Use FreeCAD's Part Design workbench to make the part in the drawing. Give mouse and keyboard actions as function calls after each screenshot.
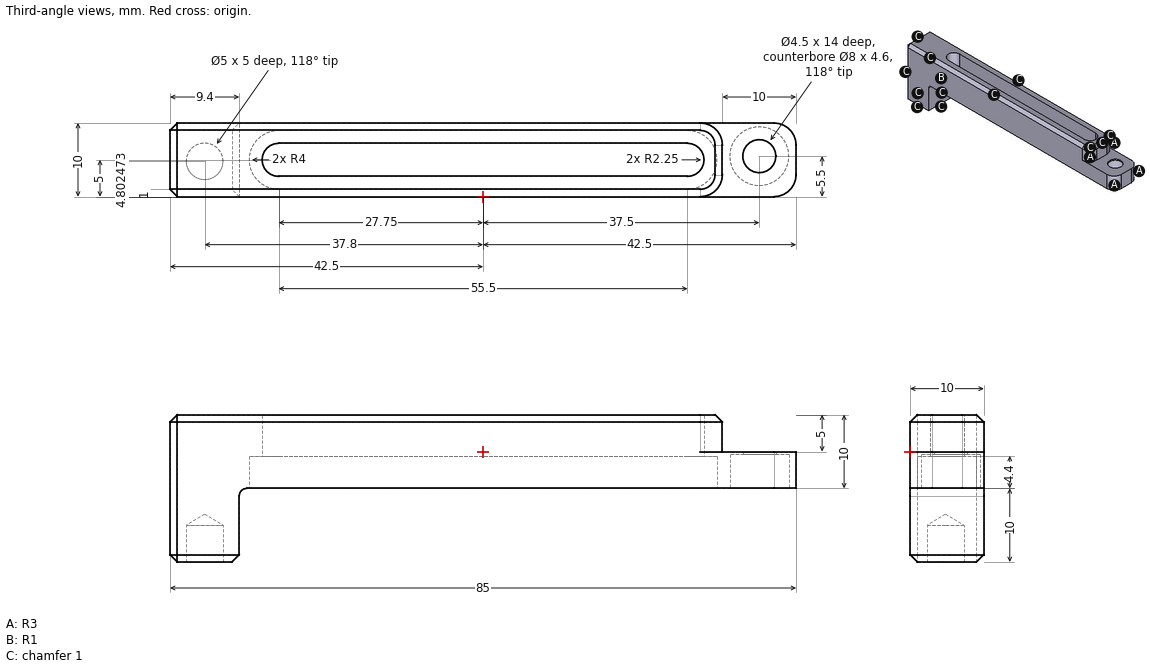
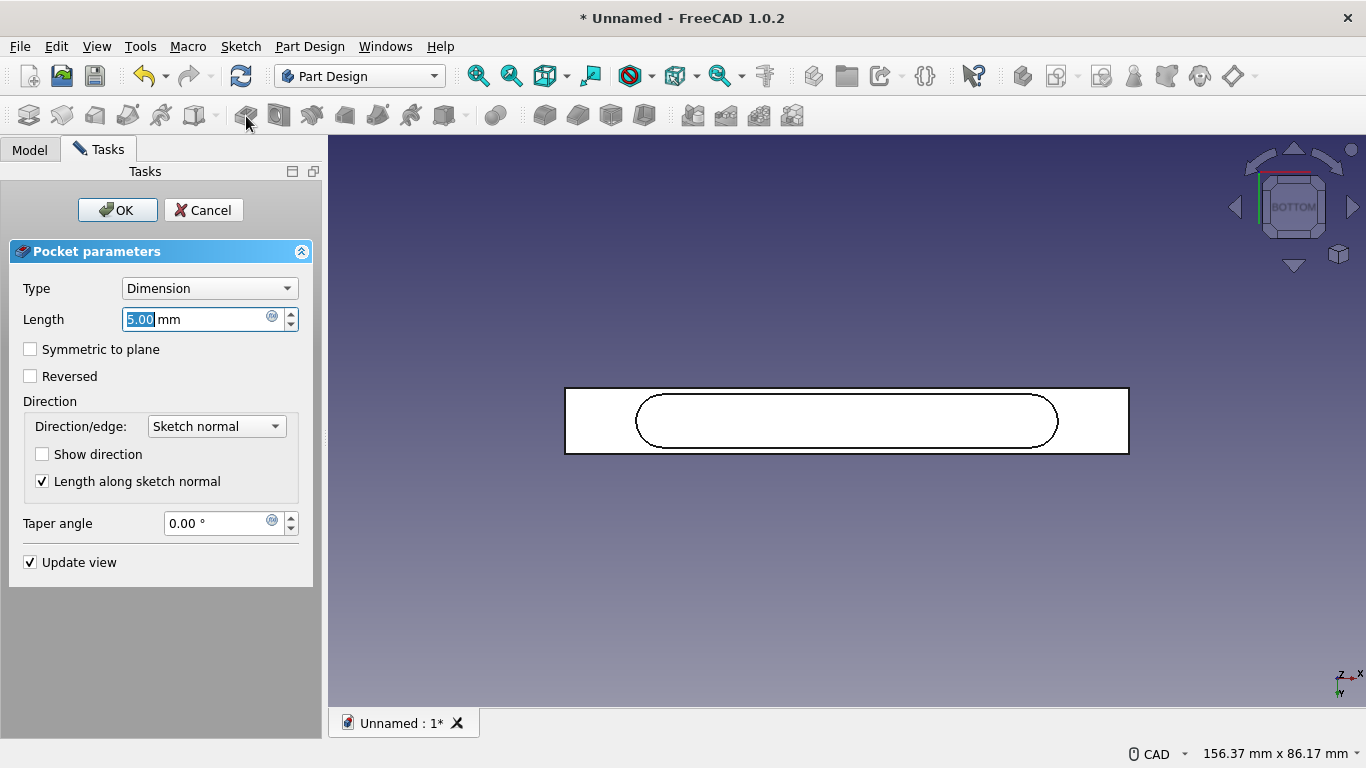
text(4.4)
key(Tab)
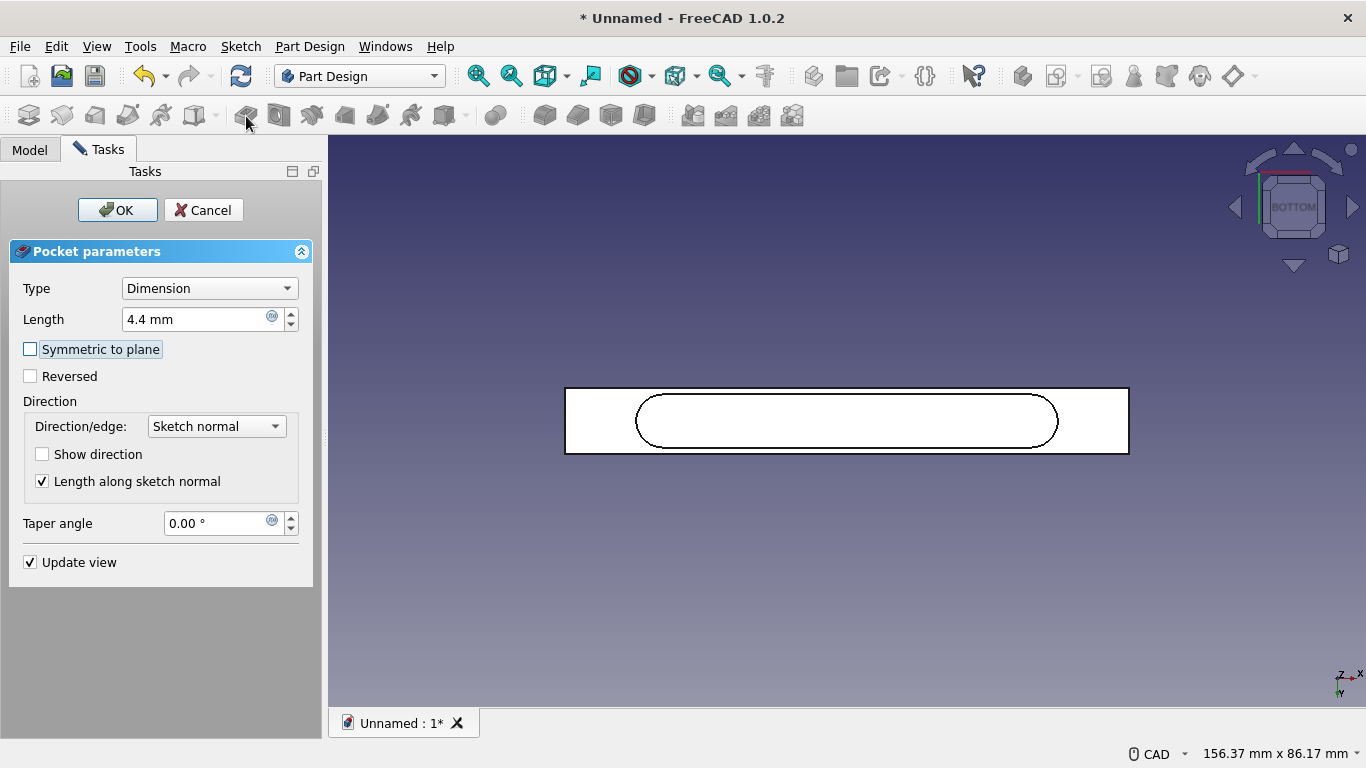
click(118, 210)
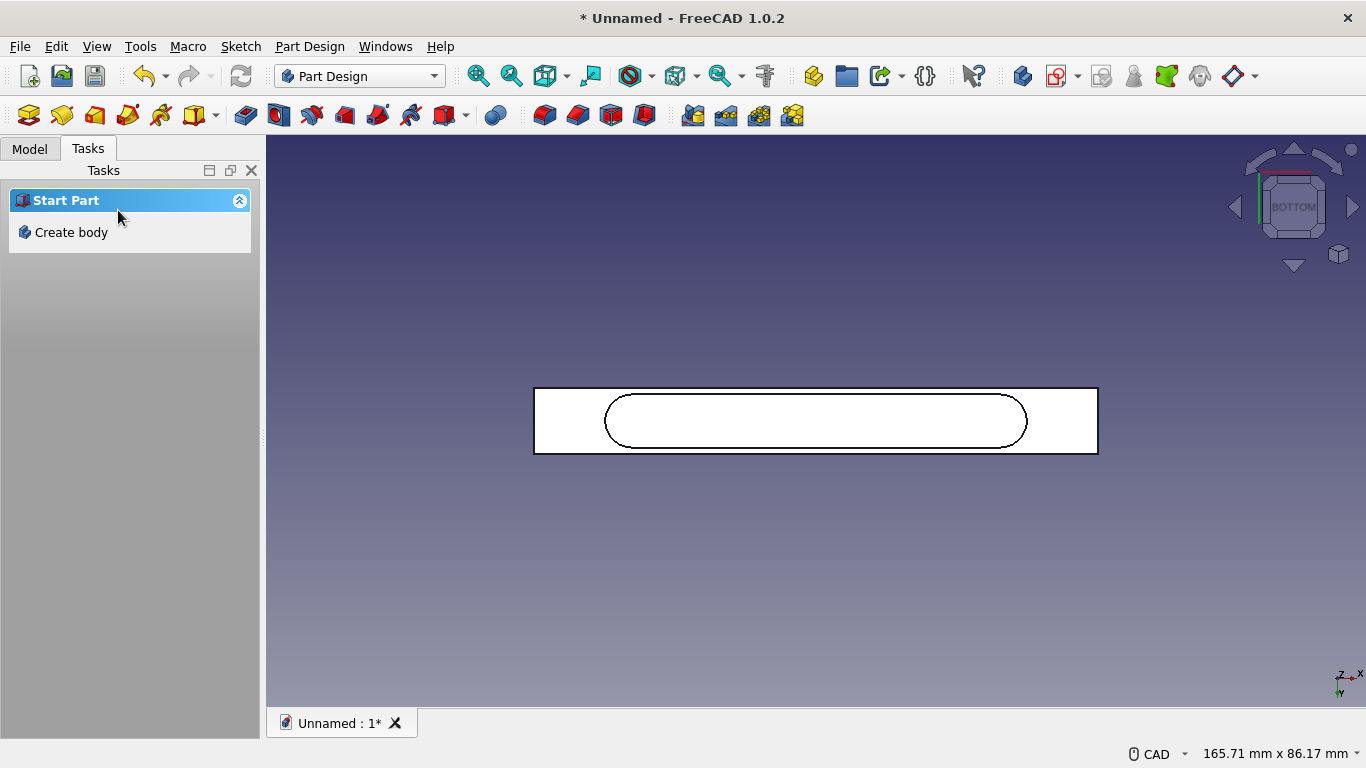
click(997, 420)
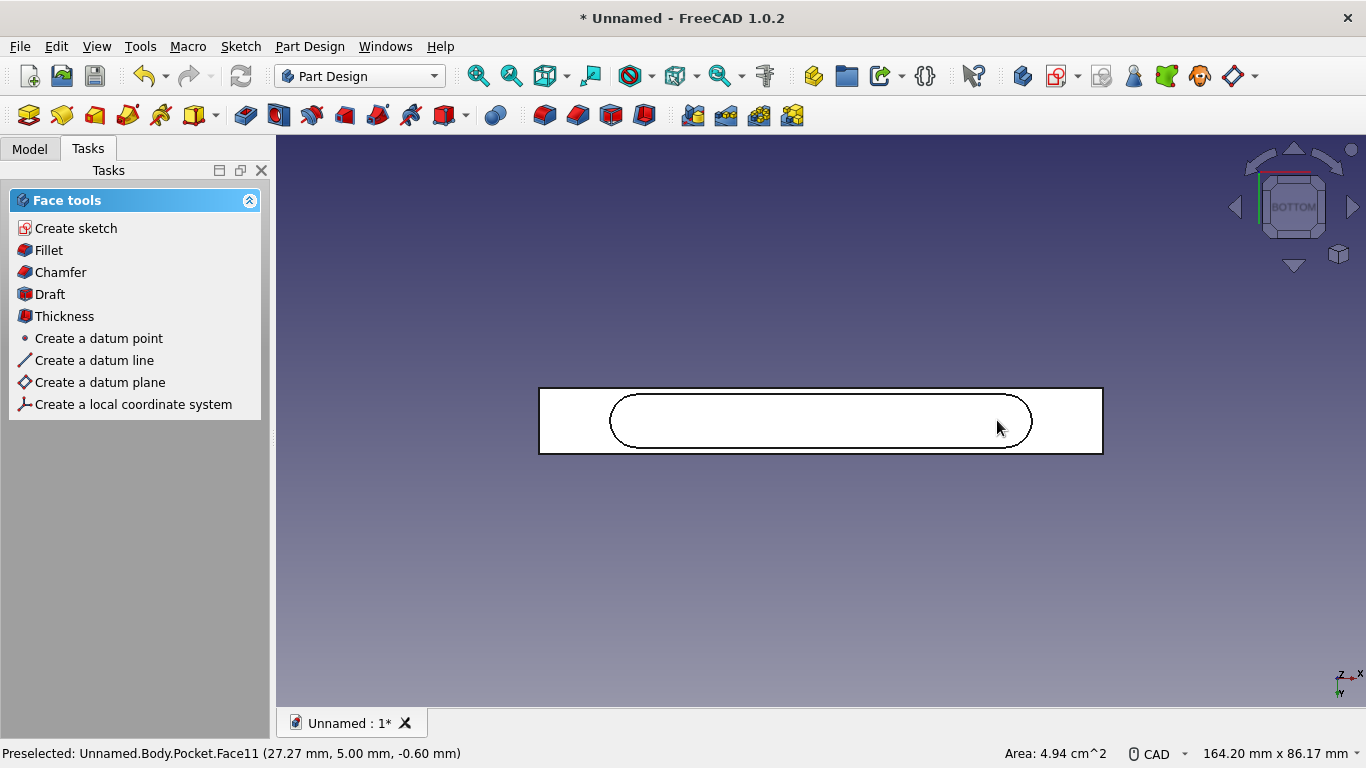
click(1056, 76)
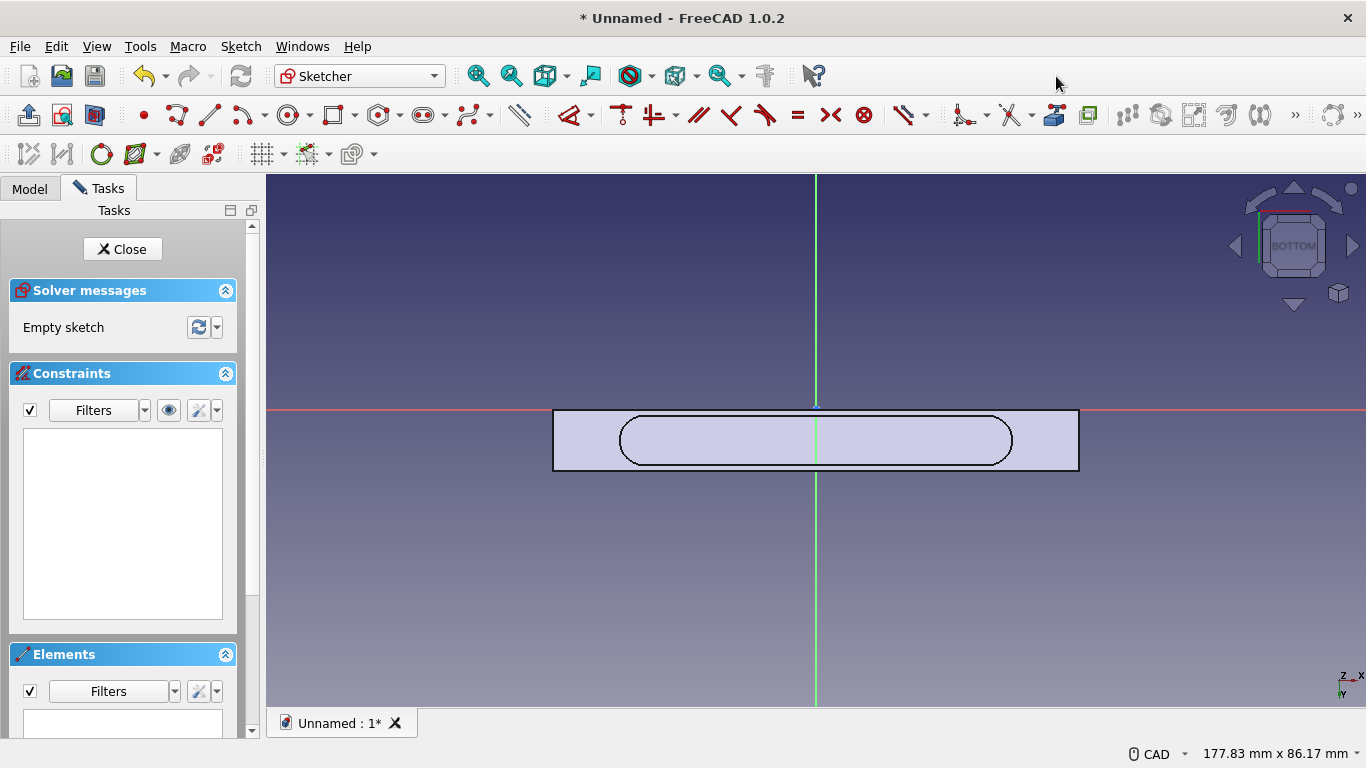
scroll(899, 422, up, 3)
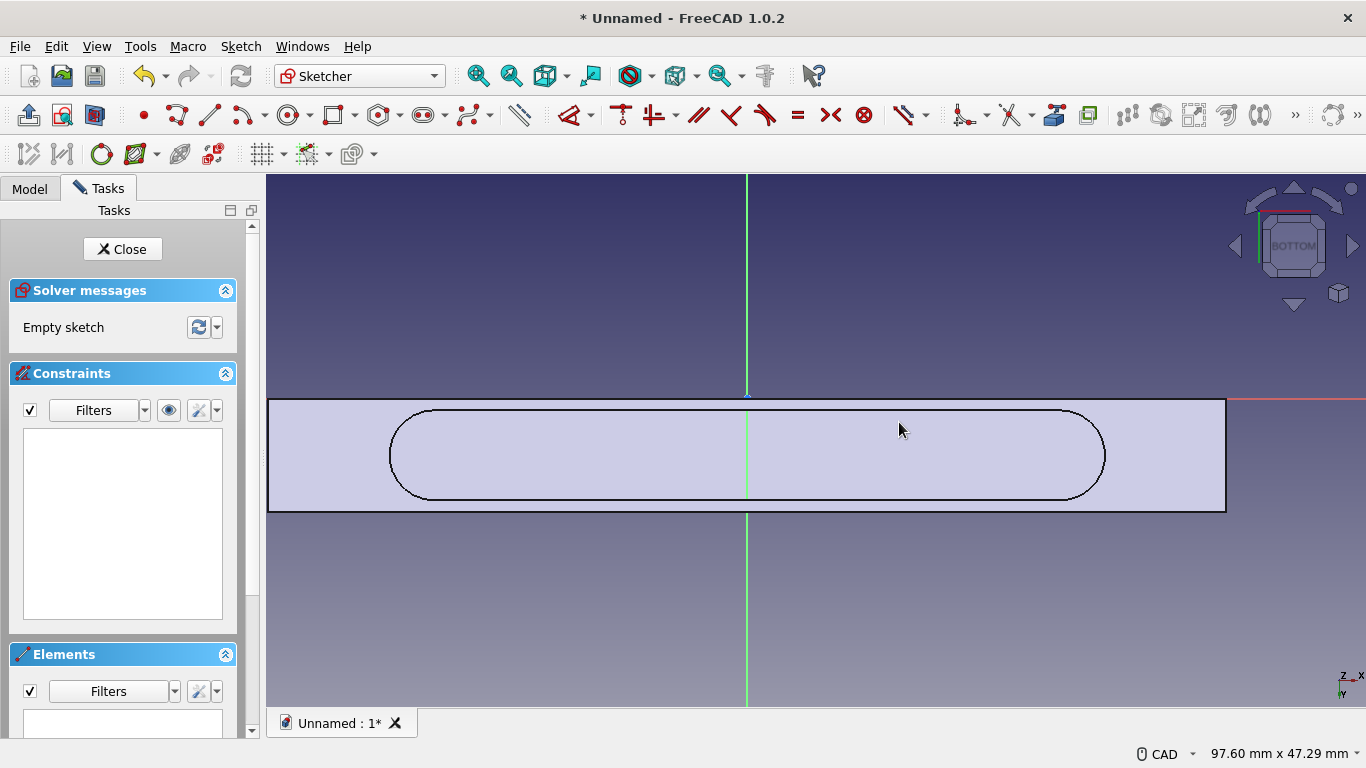
click(422, 116)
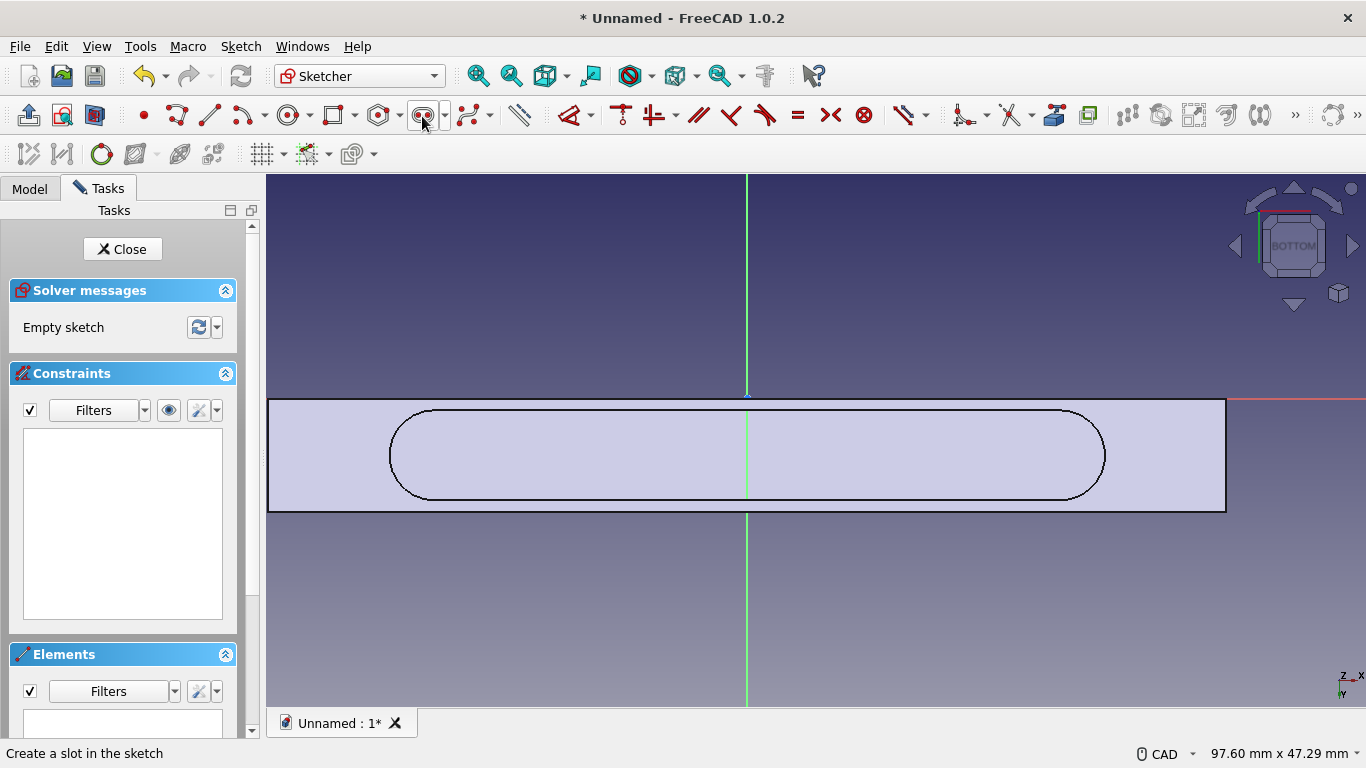
click(435, 455)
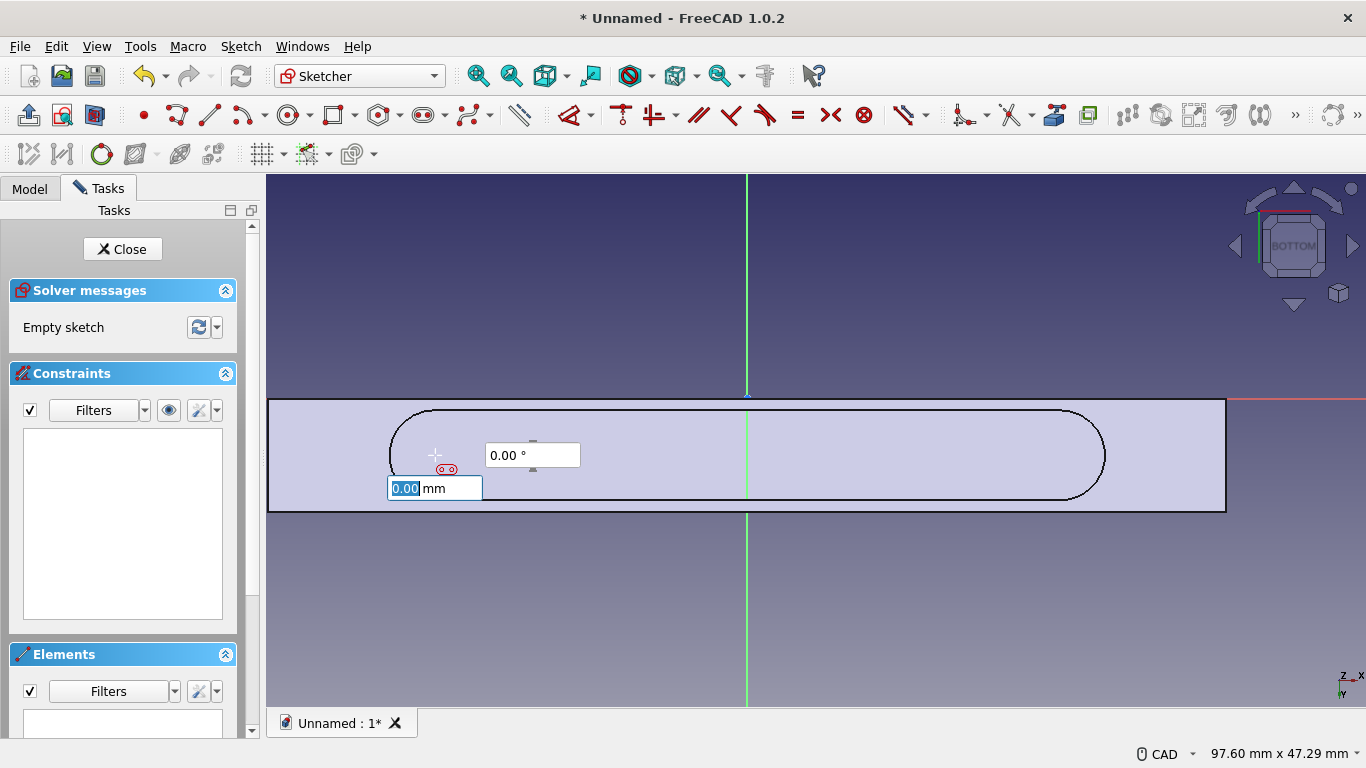
click(1060, 455)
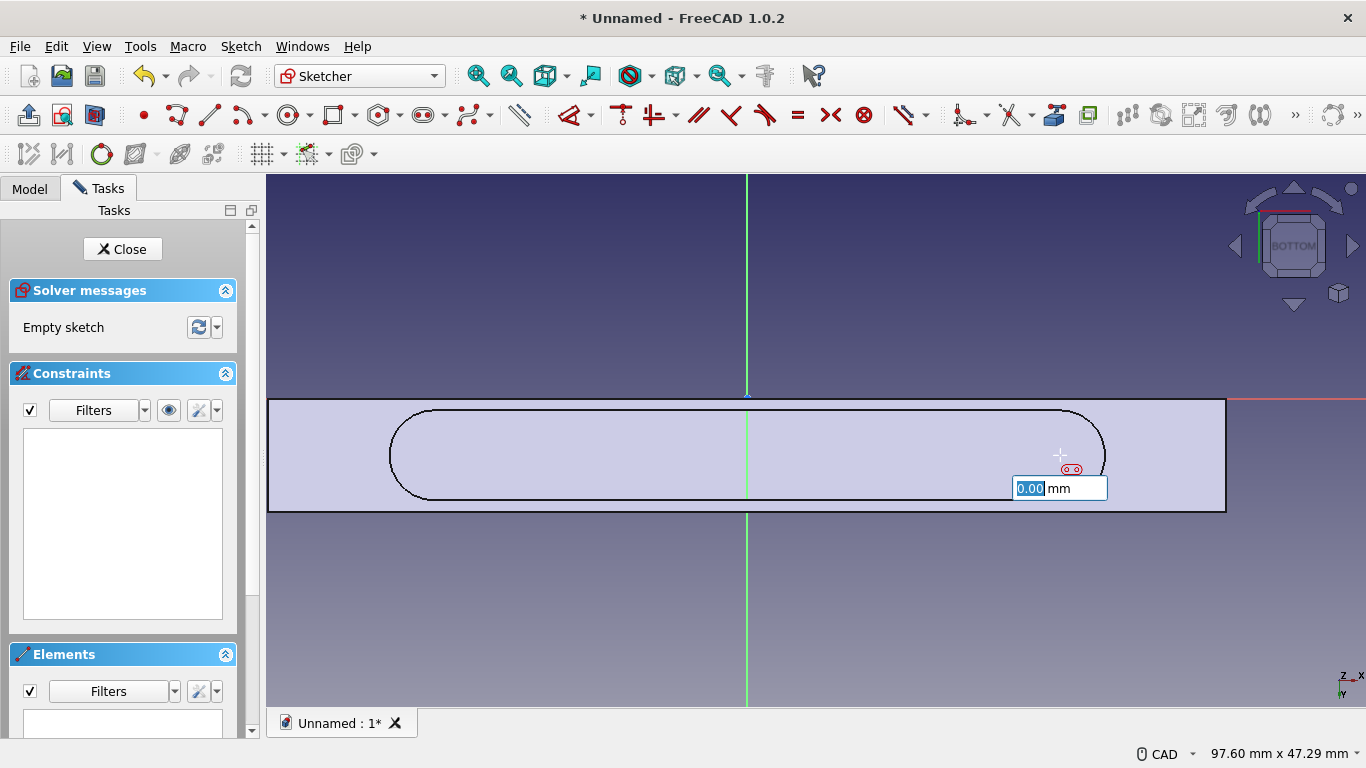
click(653, 481)
key(Escape)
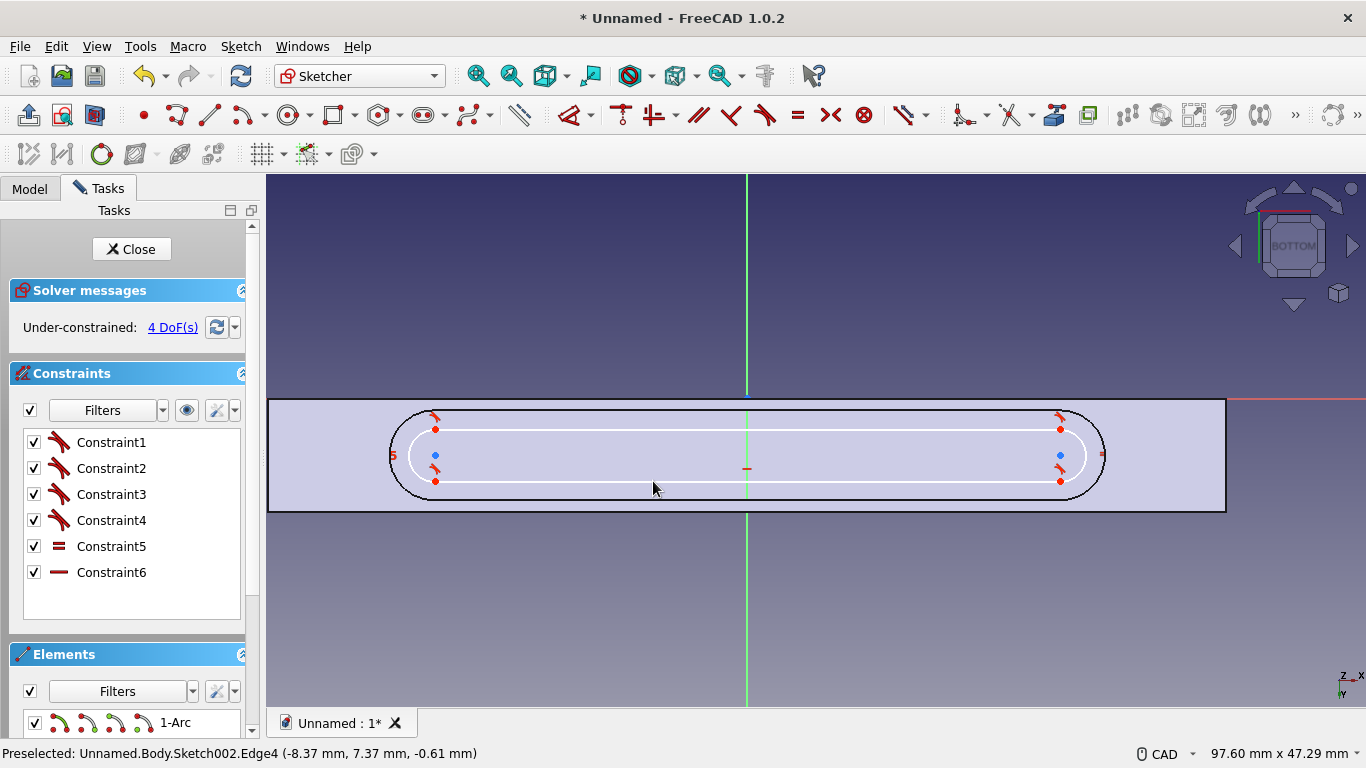
key(d)